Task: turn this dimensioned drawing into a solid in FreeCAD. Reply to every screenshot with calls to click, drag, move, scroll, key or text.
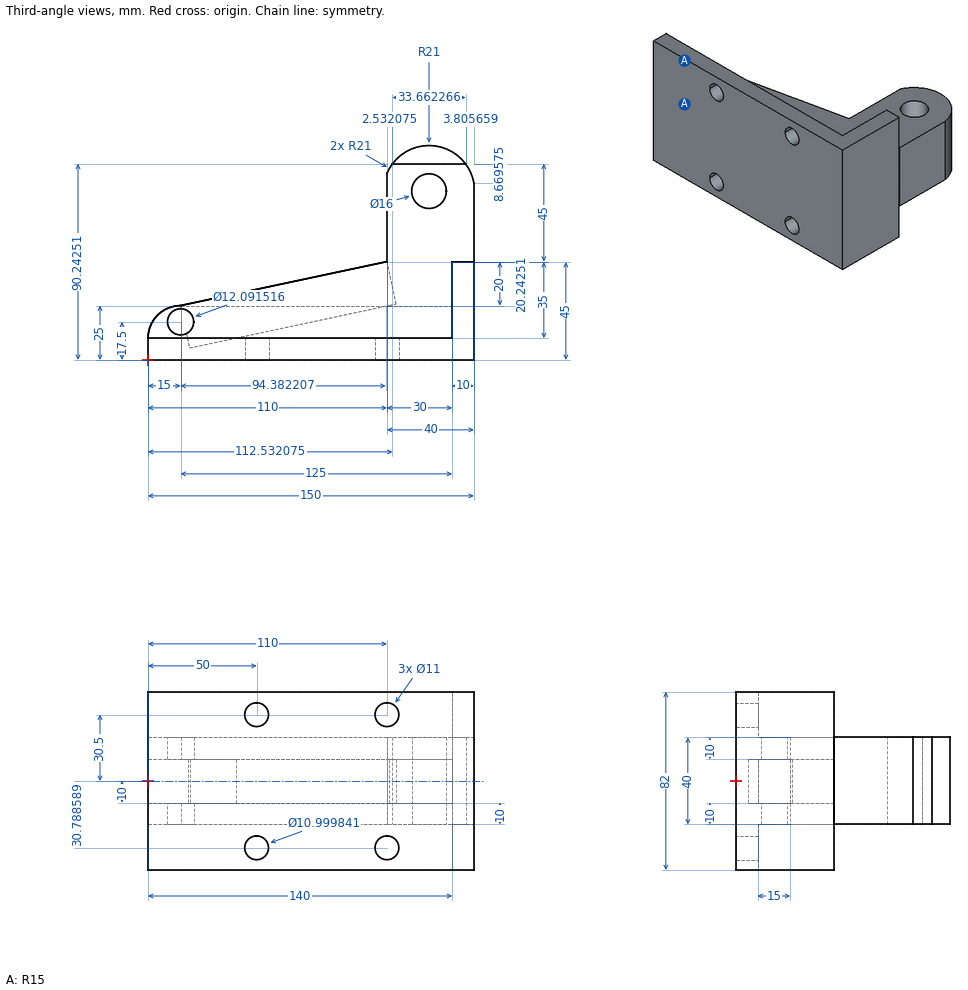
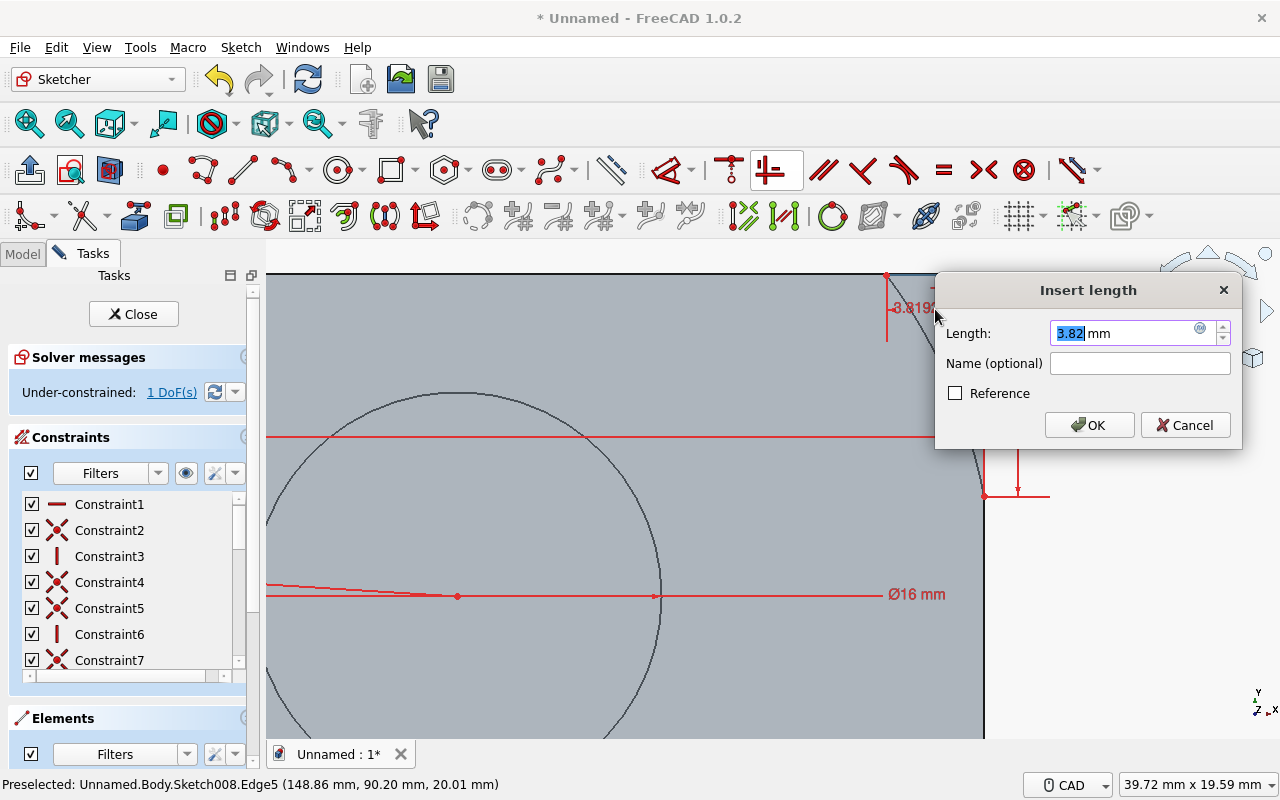
text(3.805659)
key(Return)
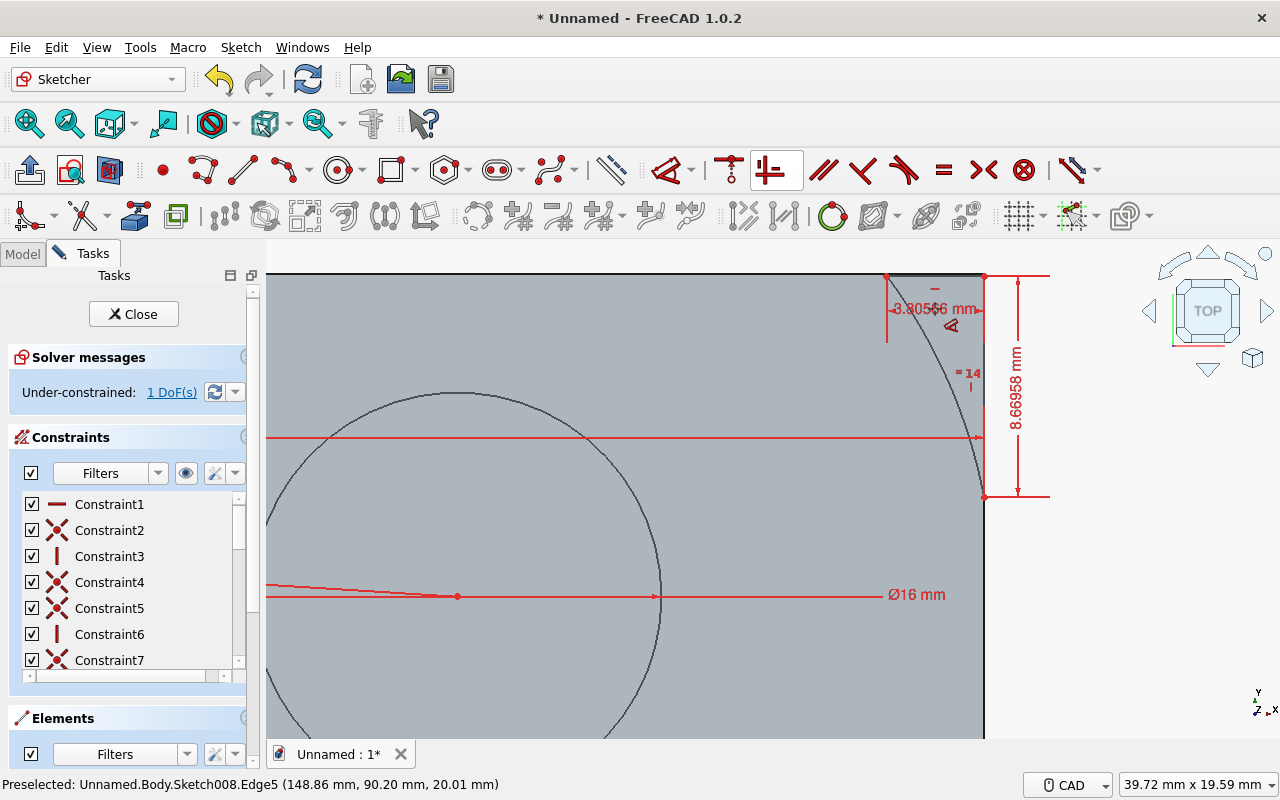
scroll(985, 431, down, 3)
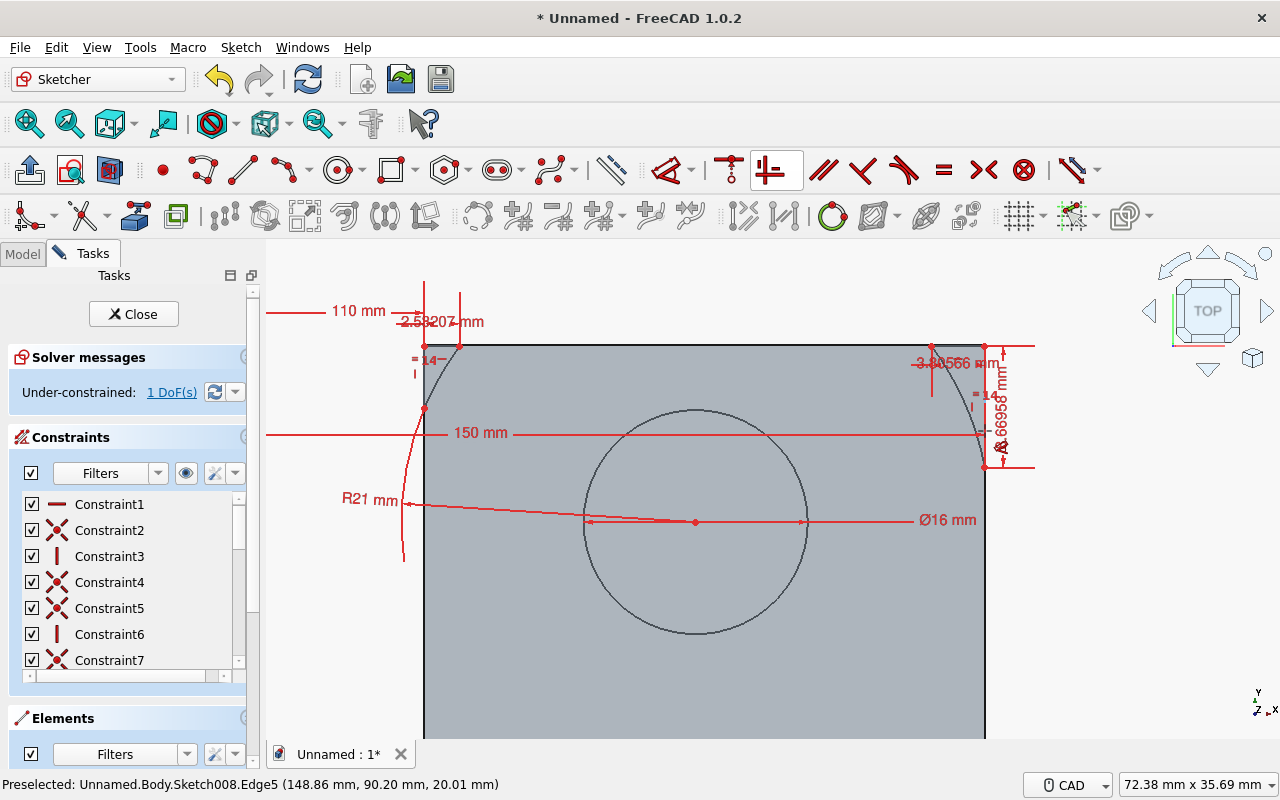
click(460, 346)
click(494, 529)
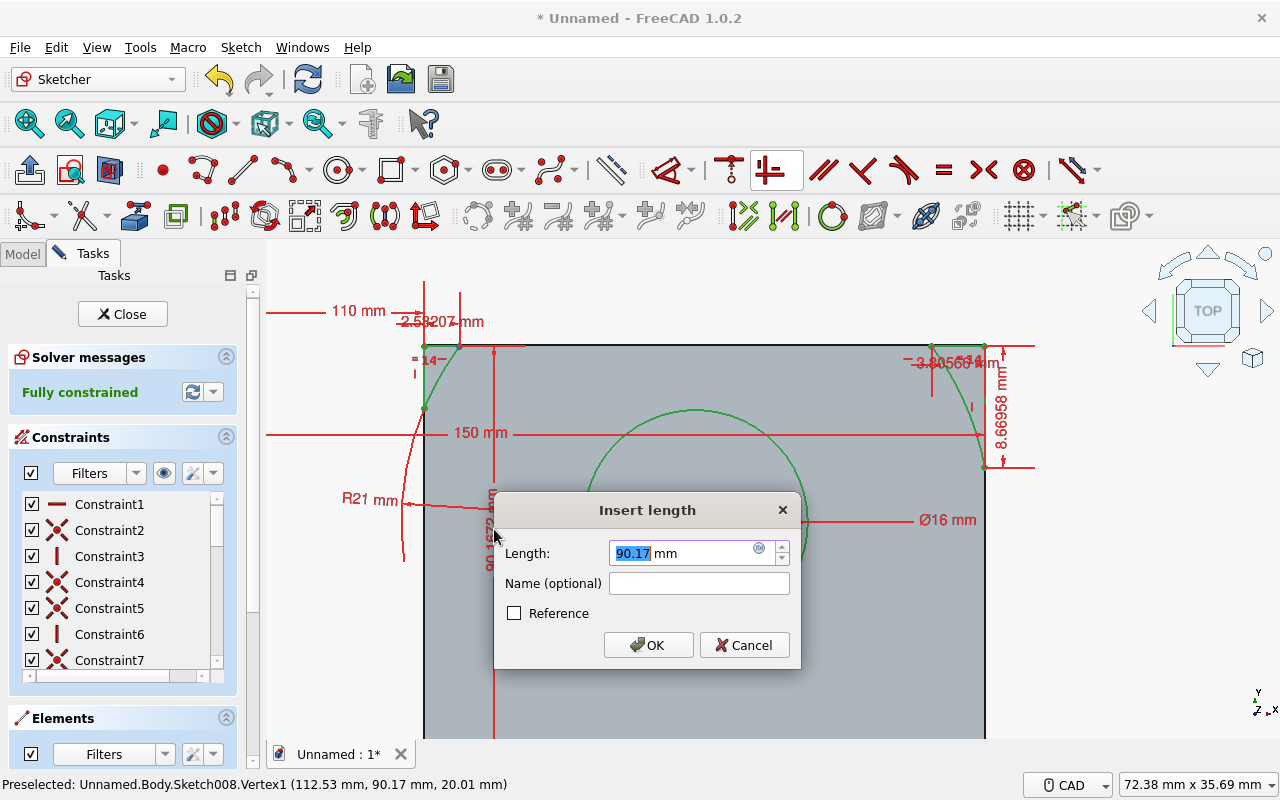
text(90.24251)
key(Return)
key(Escape)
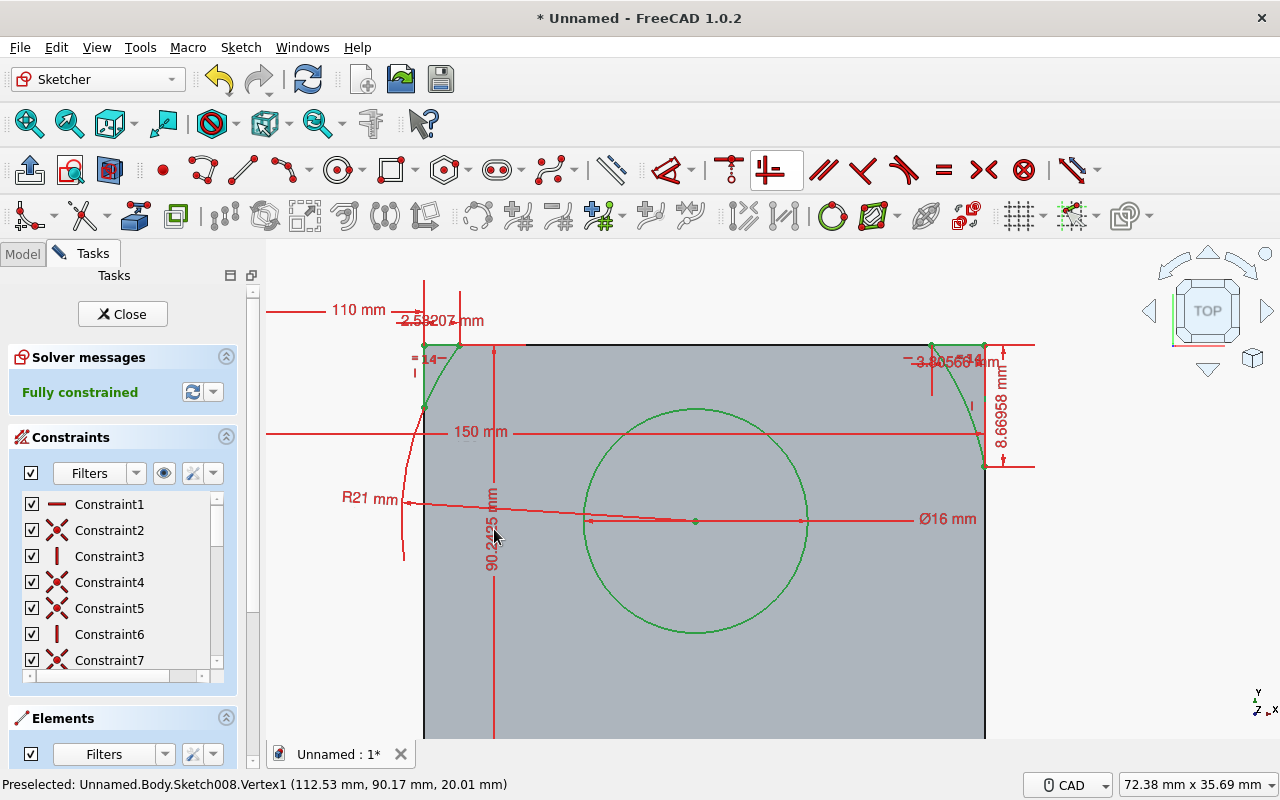
click(123, 314)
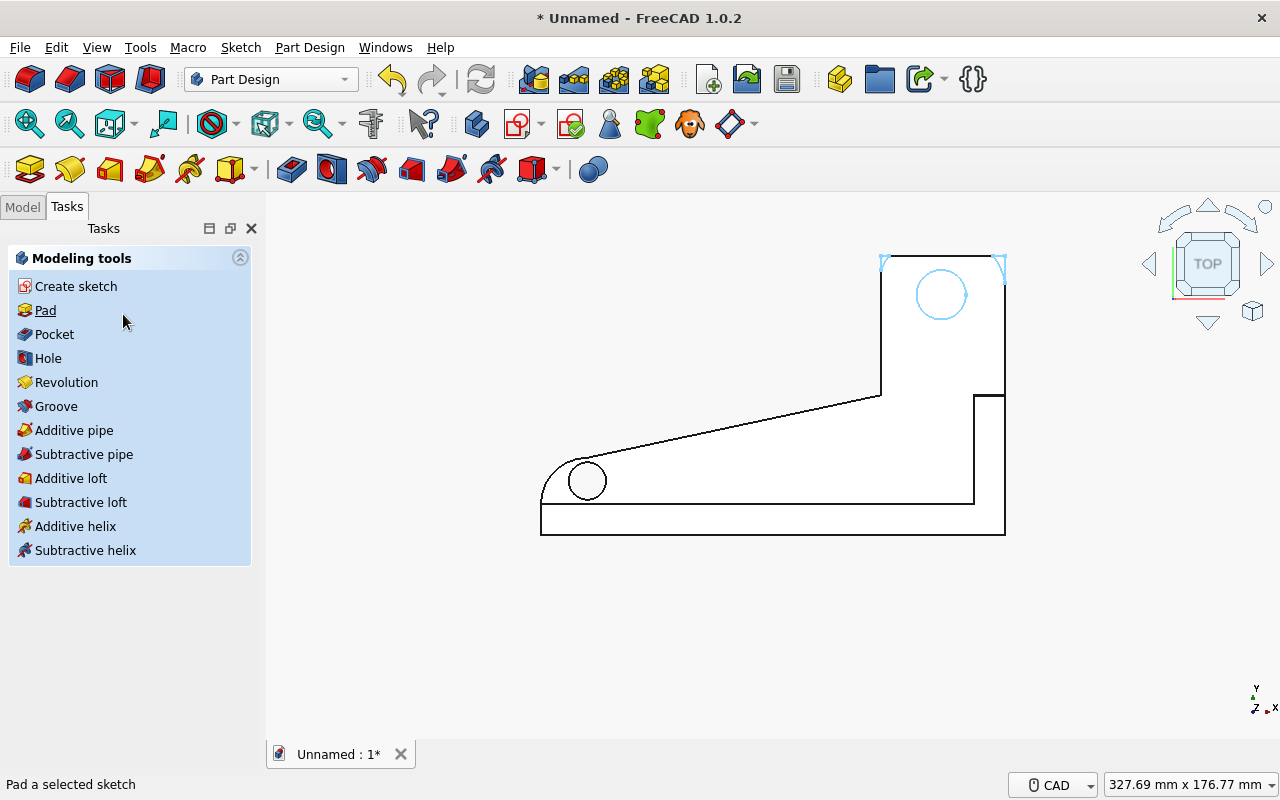
click(292, 170)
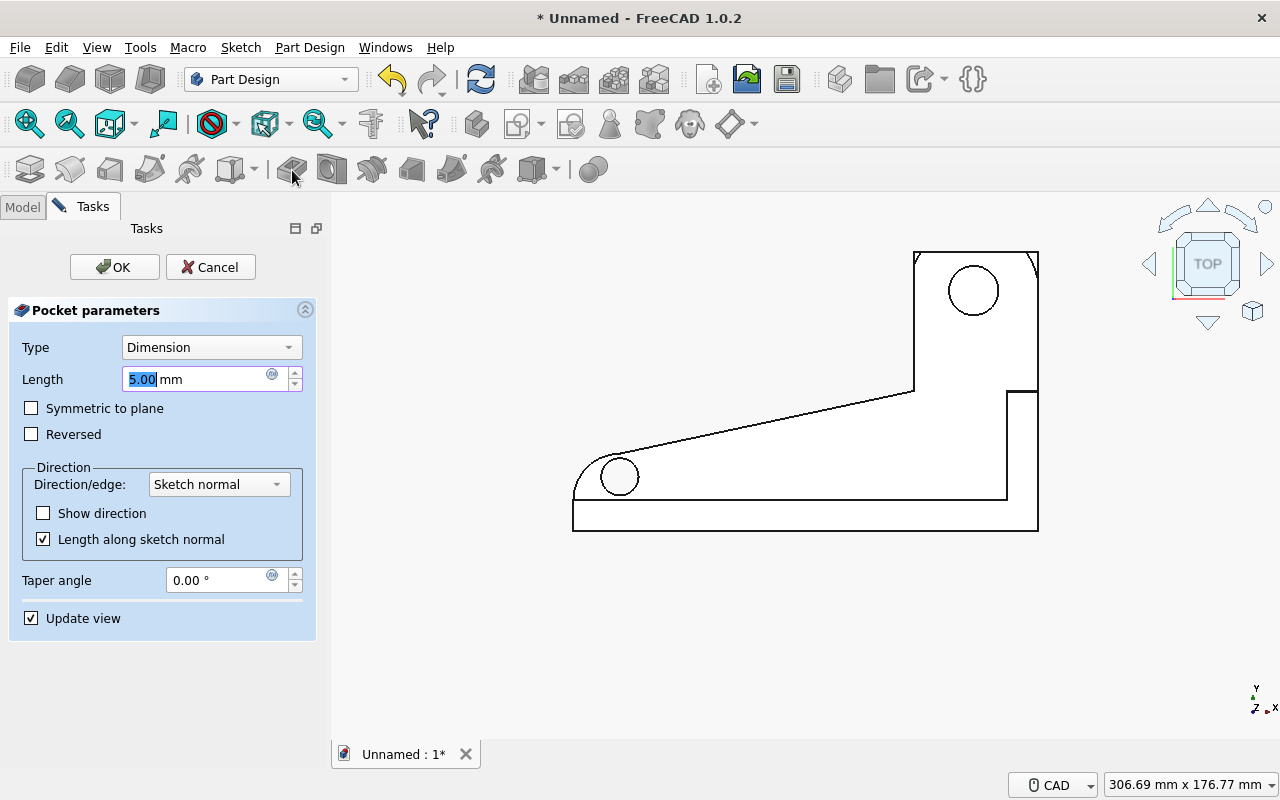
text(40)
key(Tab)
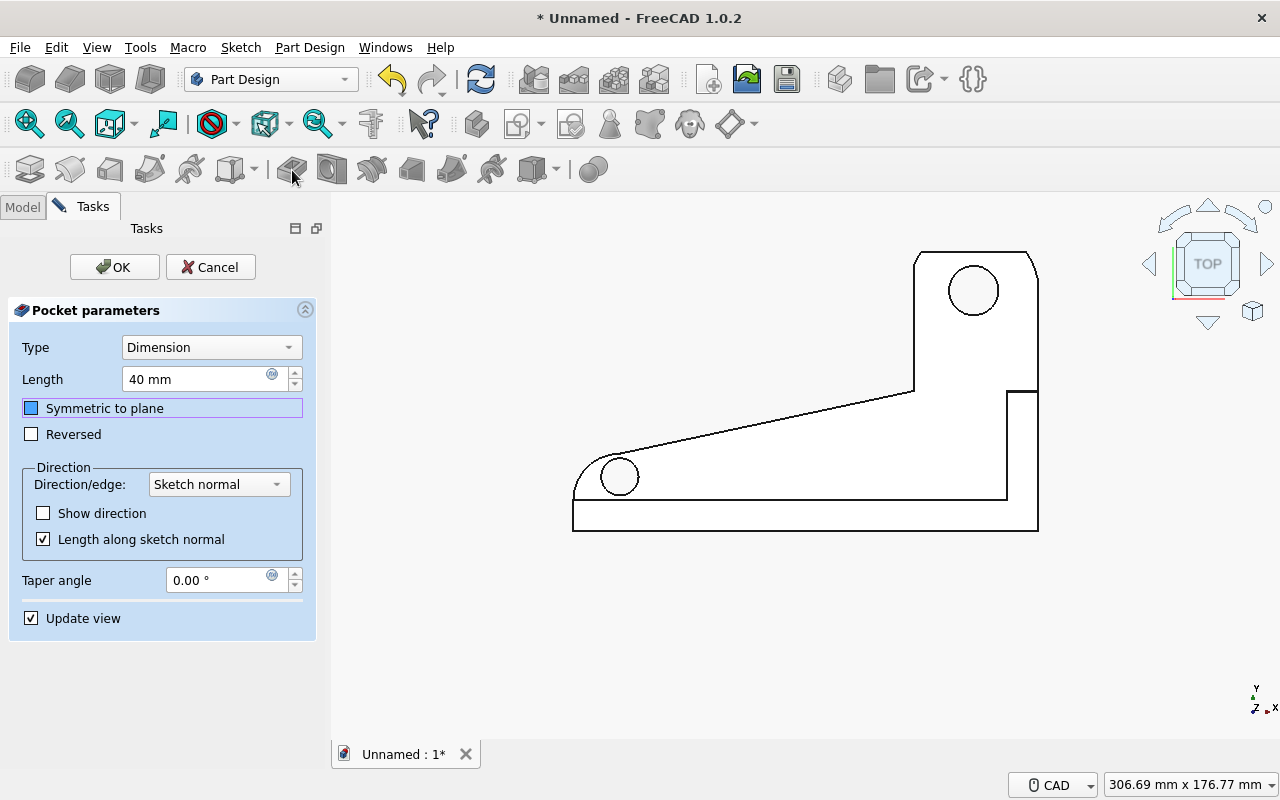
click(115, 267)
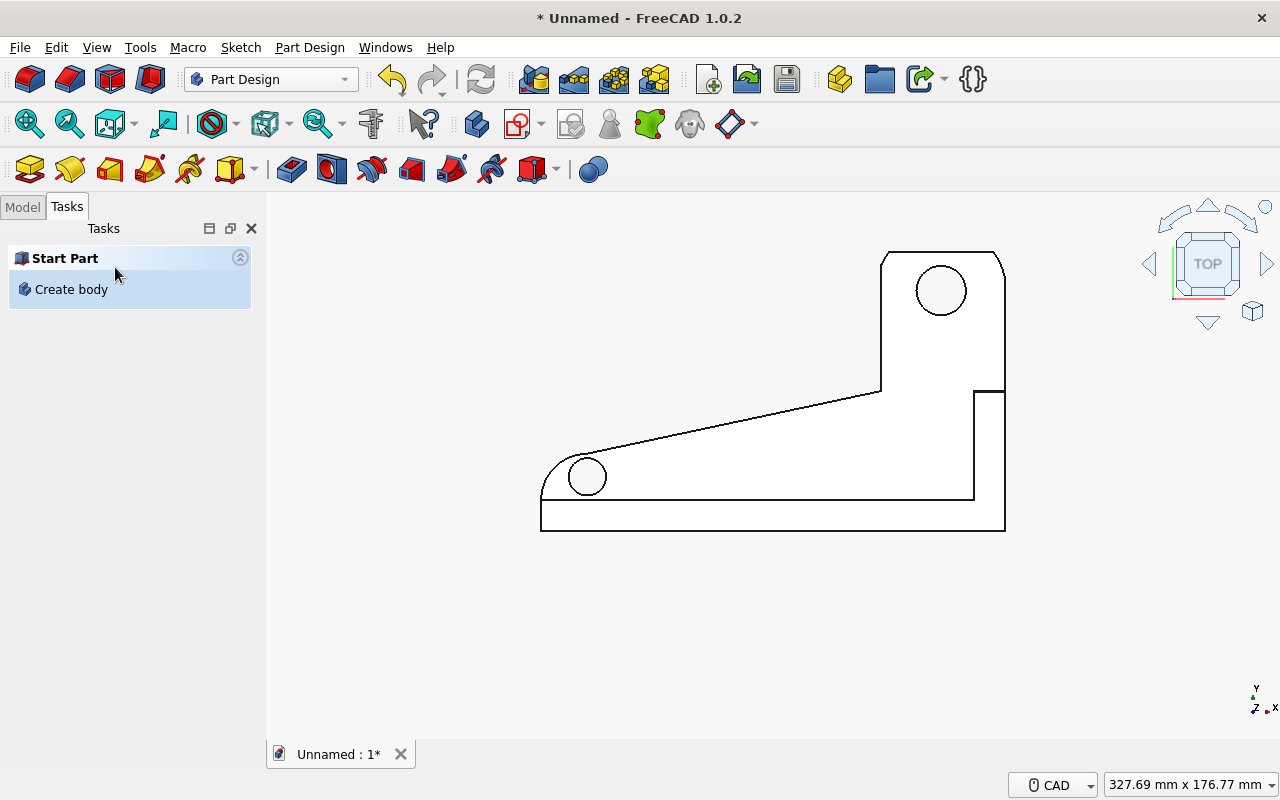
click(906, 446)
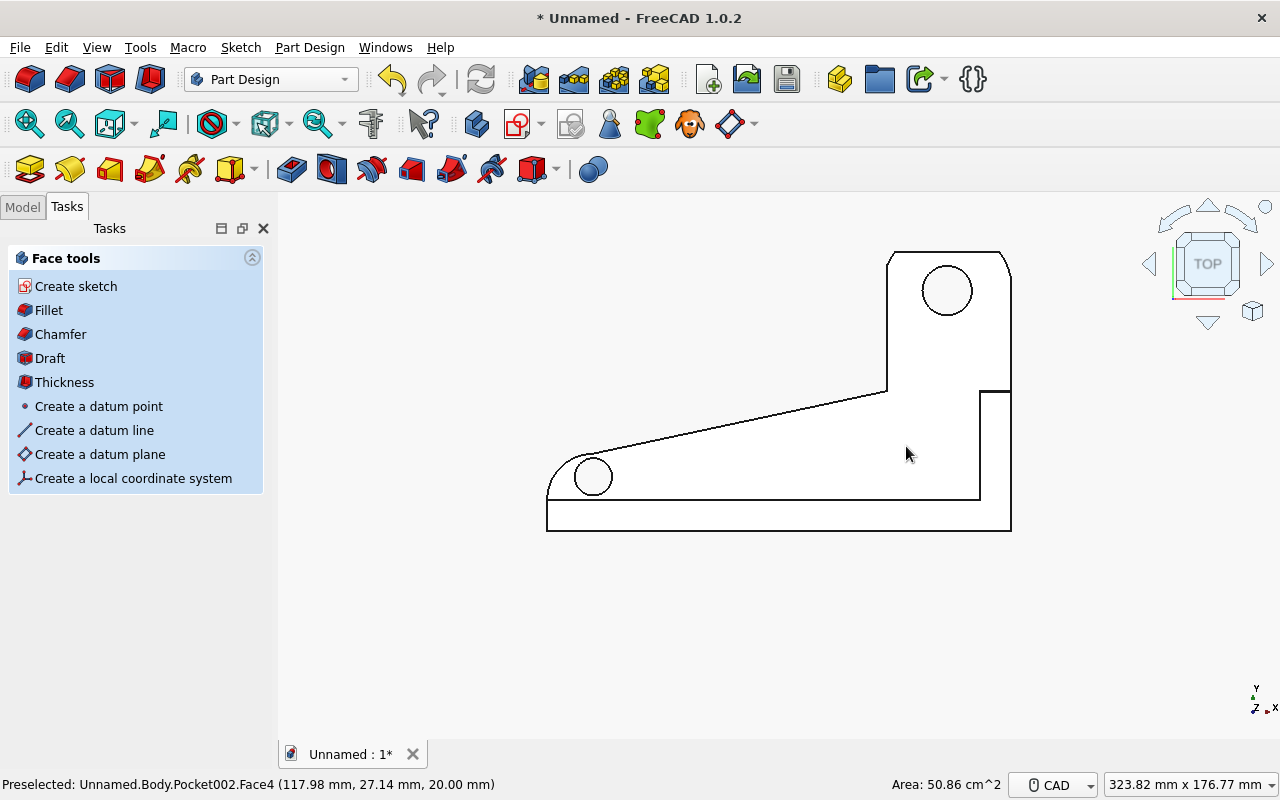
click(518, 124)